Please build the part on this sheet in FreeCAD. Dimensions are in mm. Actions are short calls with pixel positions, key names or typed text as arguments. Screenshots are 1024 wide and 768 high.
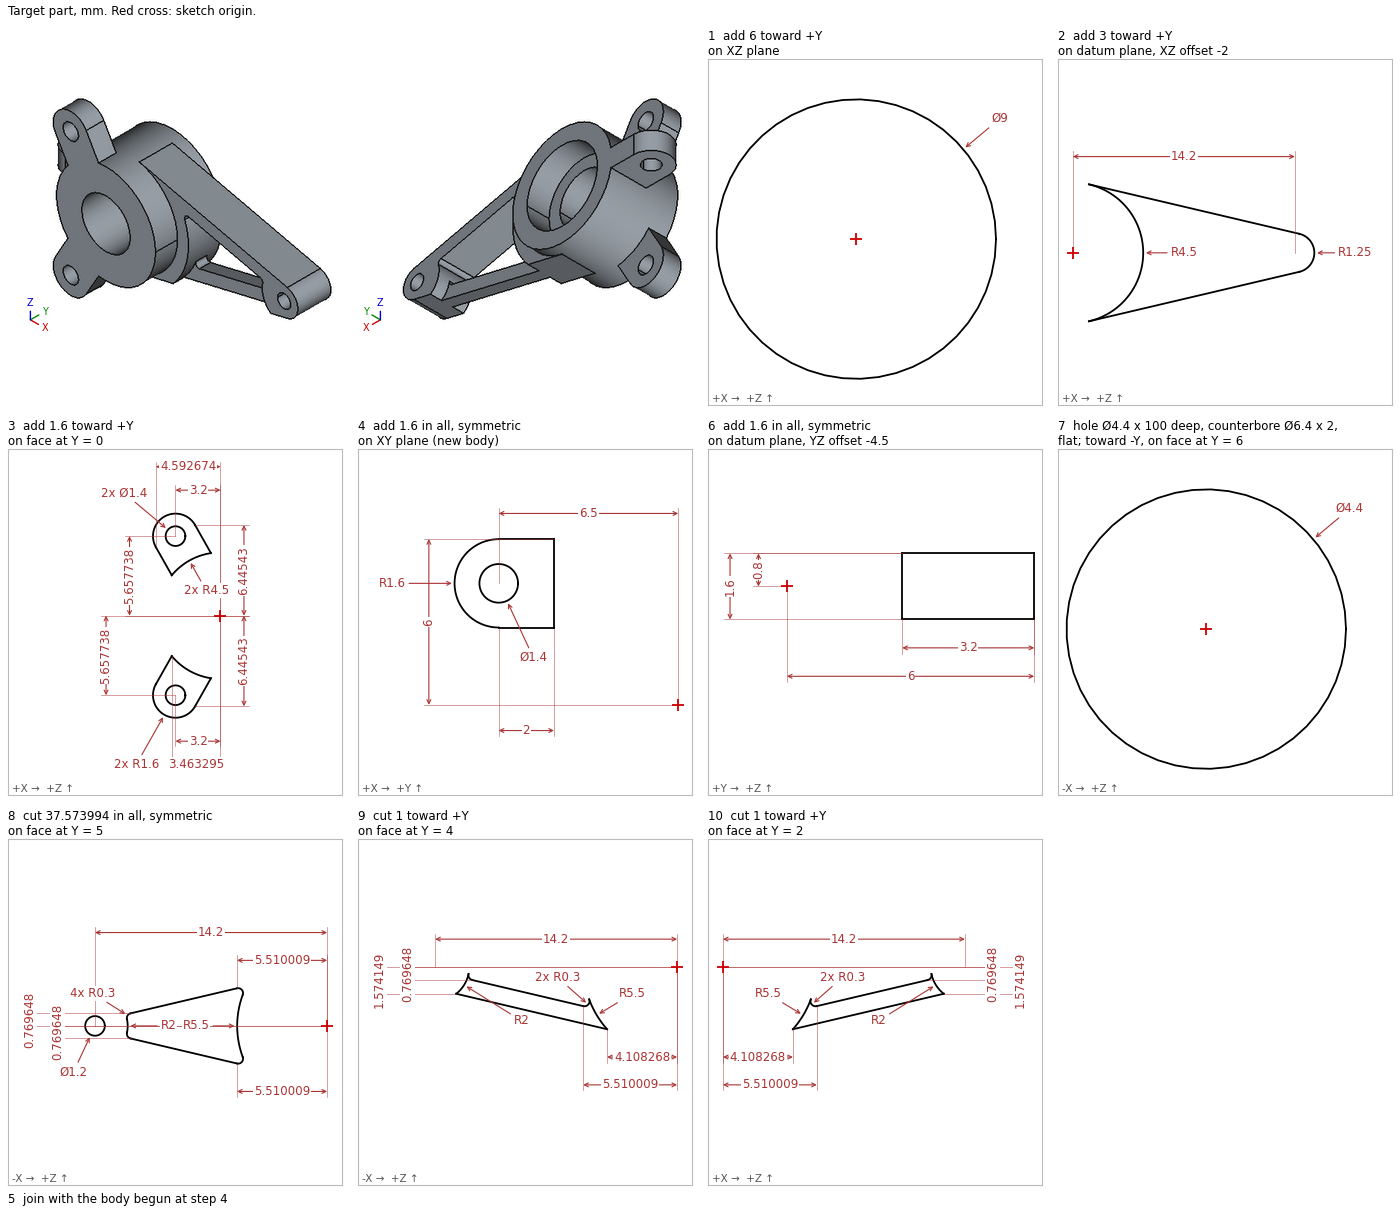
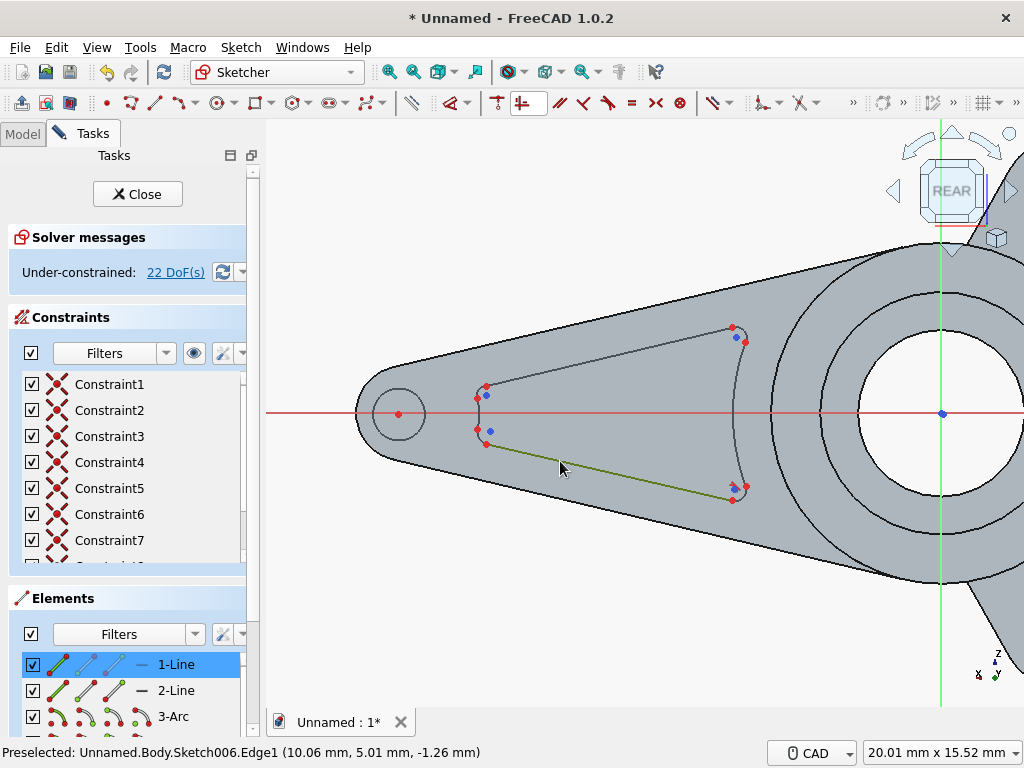
scroll(480, 439, up, 3)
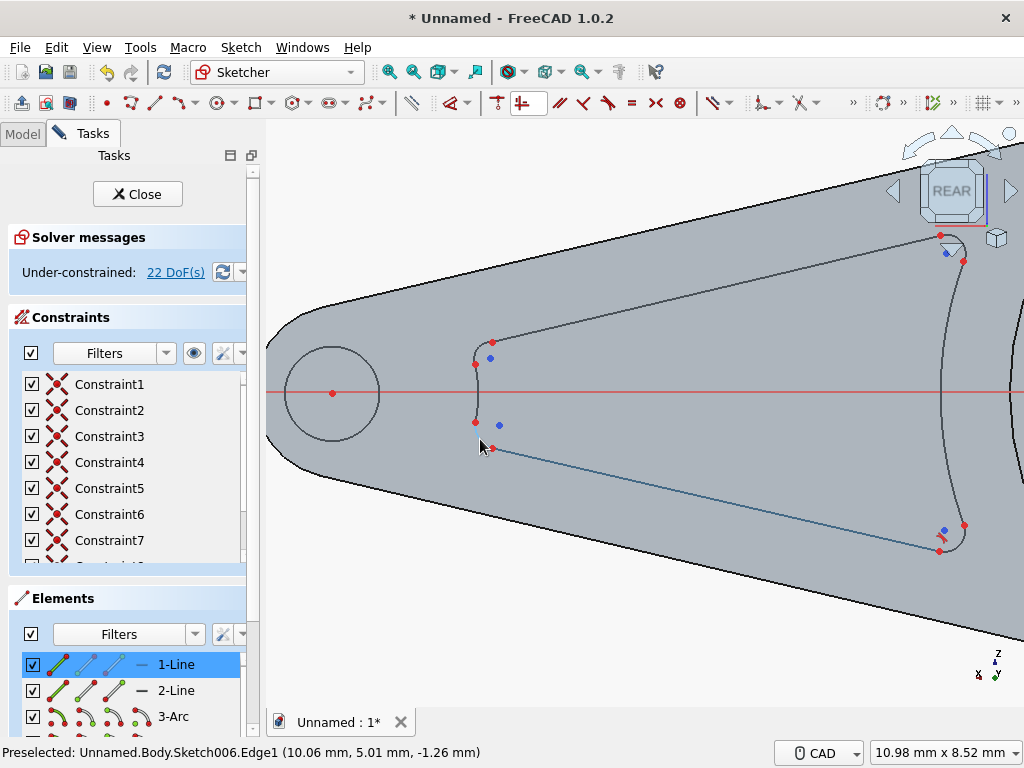
click(479, 438)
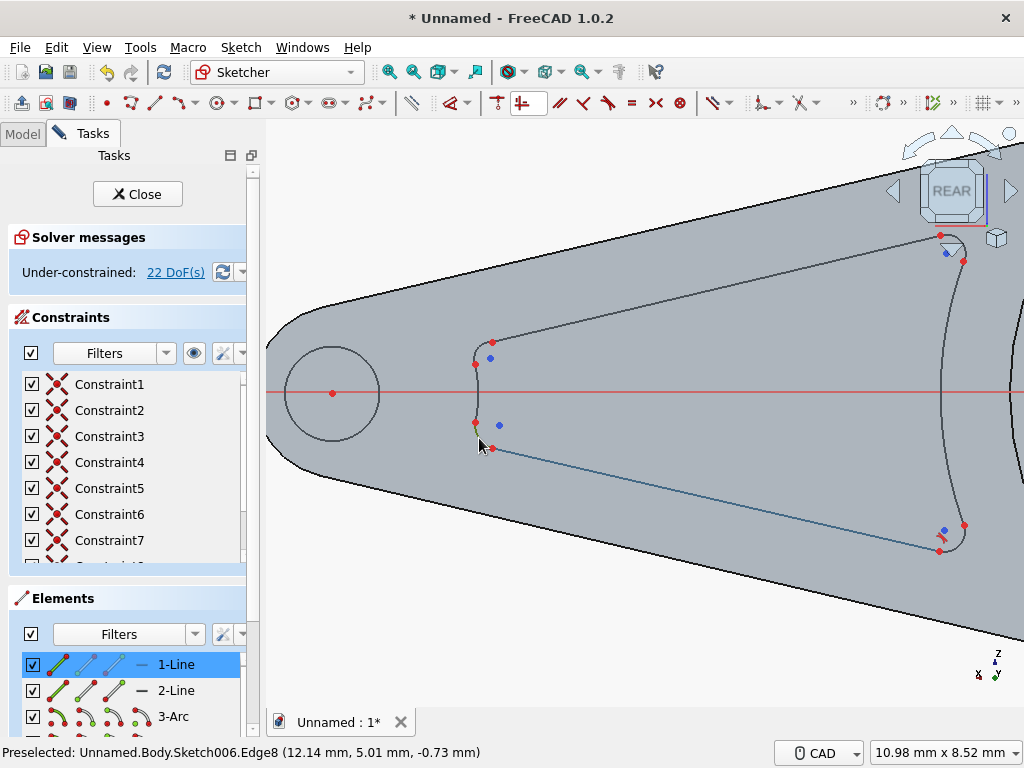
key(t)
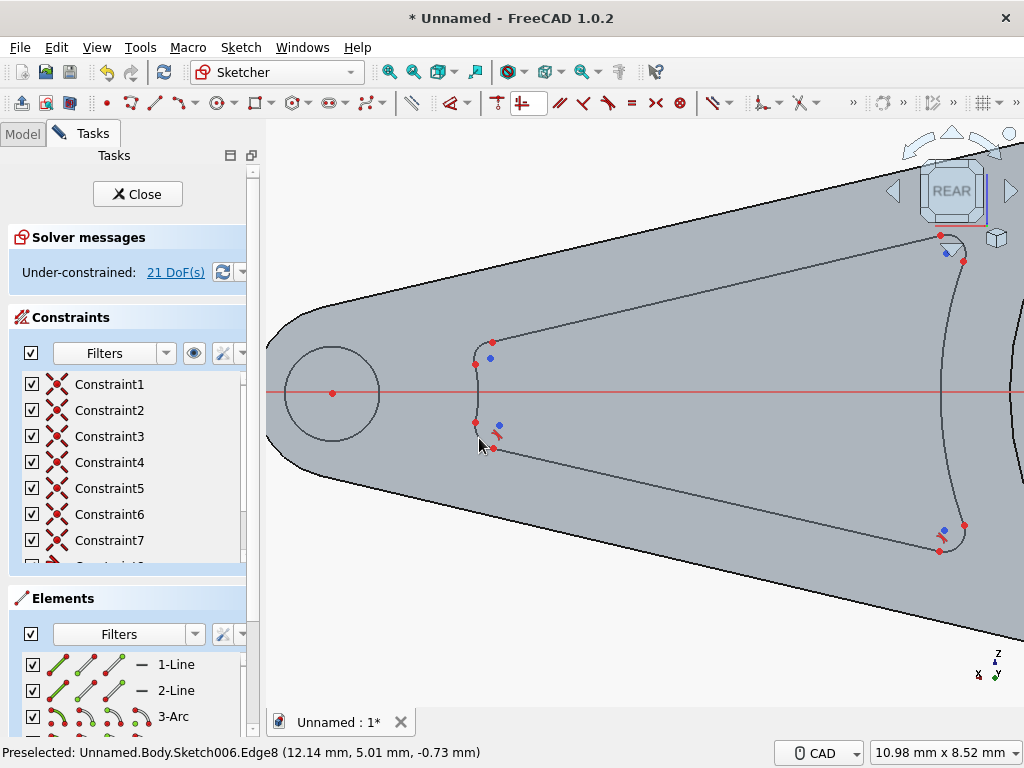
click(806, 268)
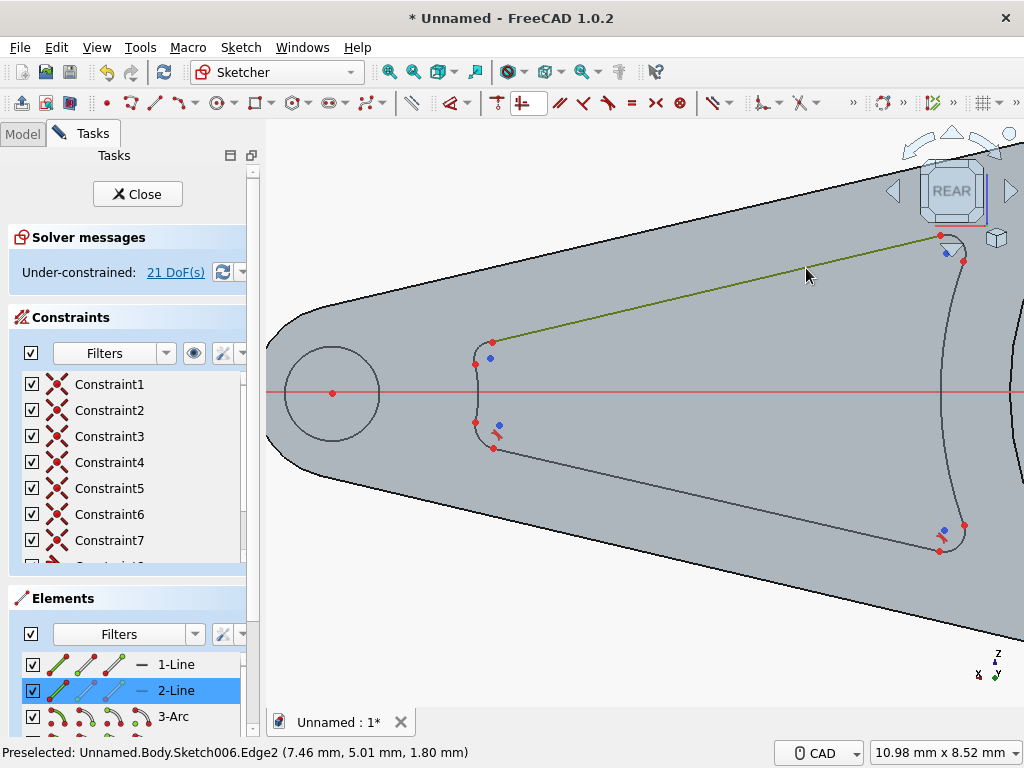
scroll(441, 425, down, 5)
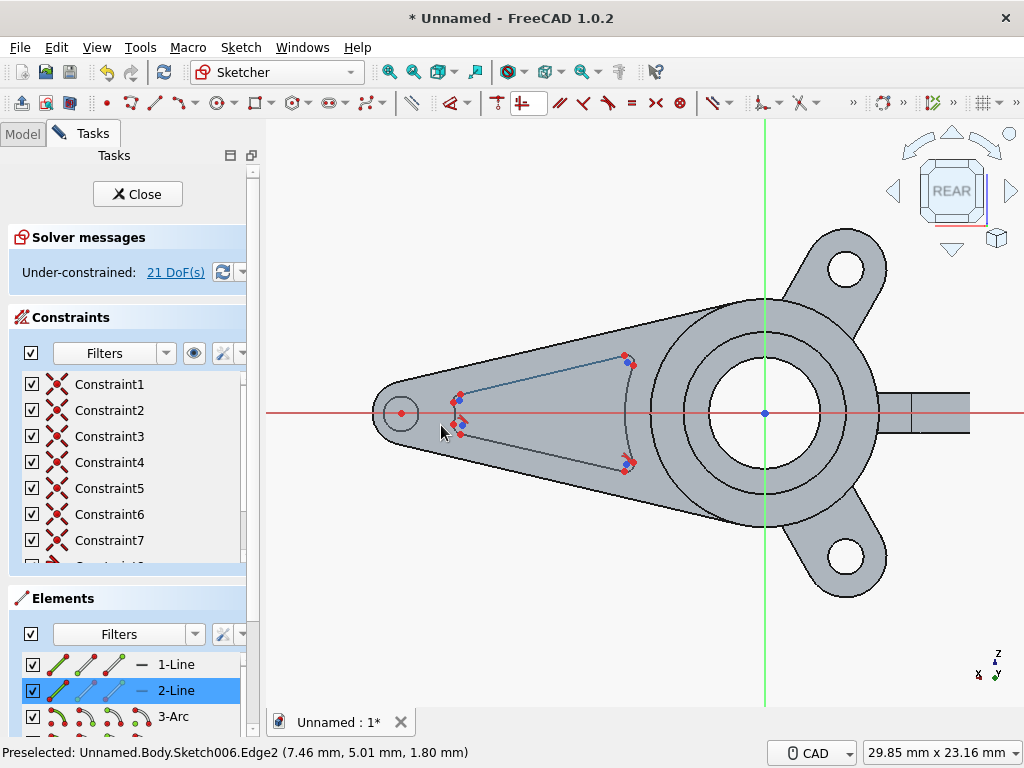
scroll(634, 361, up, 6)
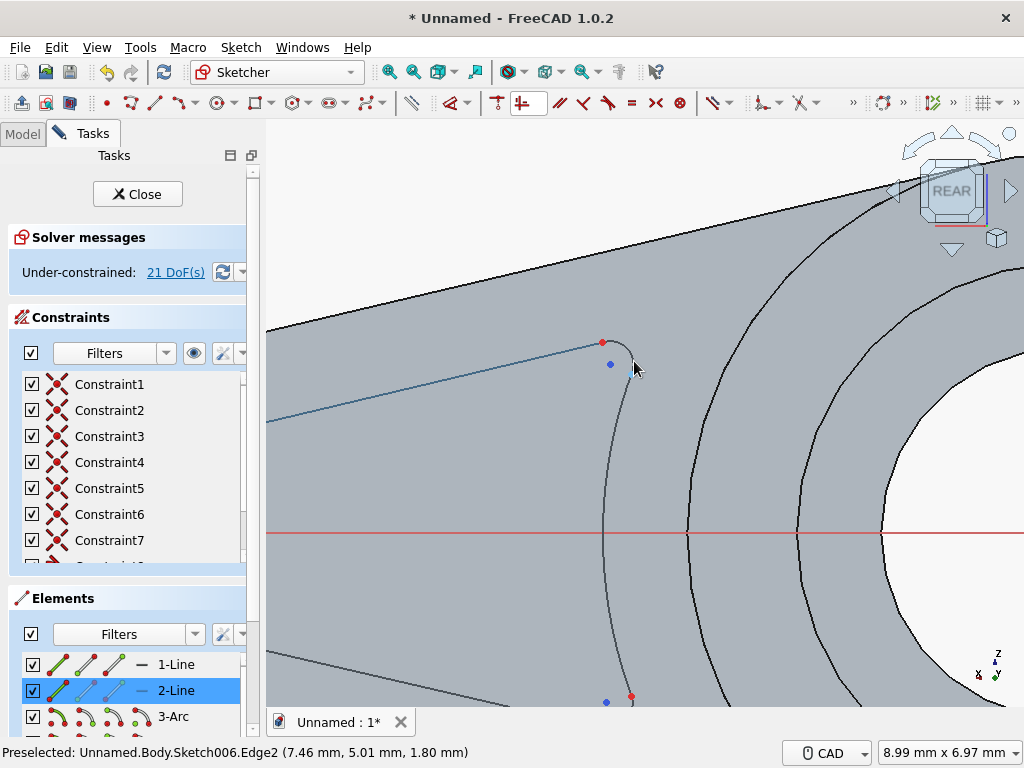
click(633, 359)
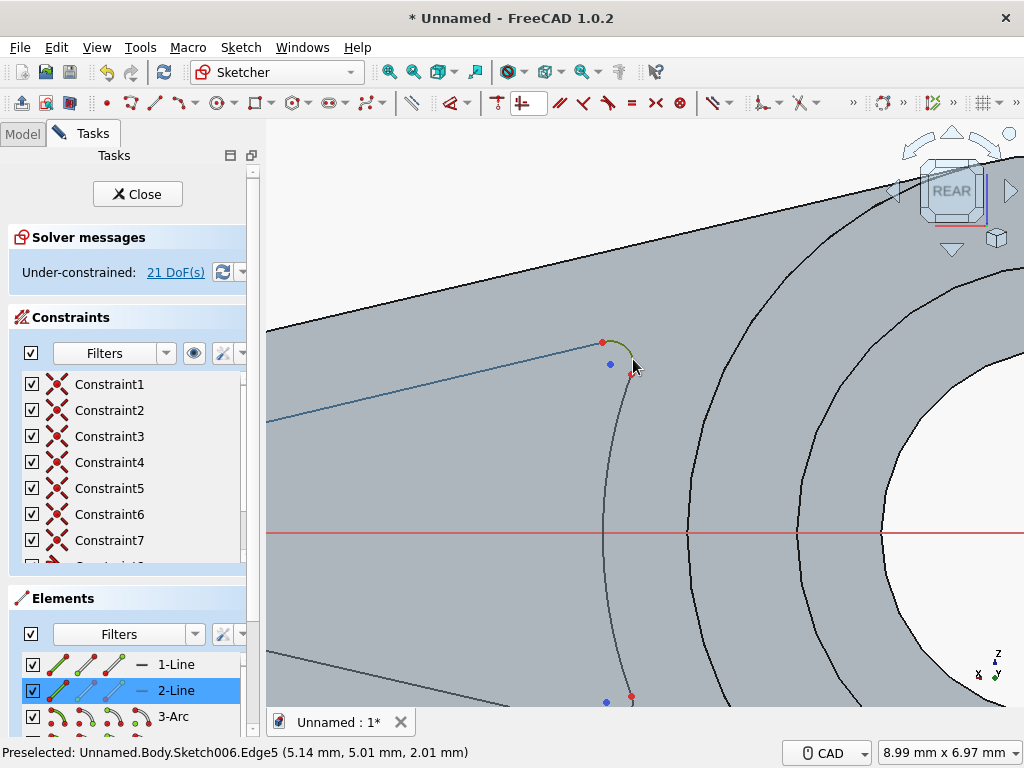
click(608, 104)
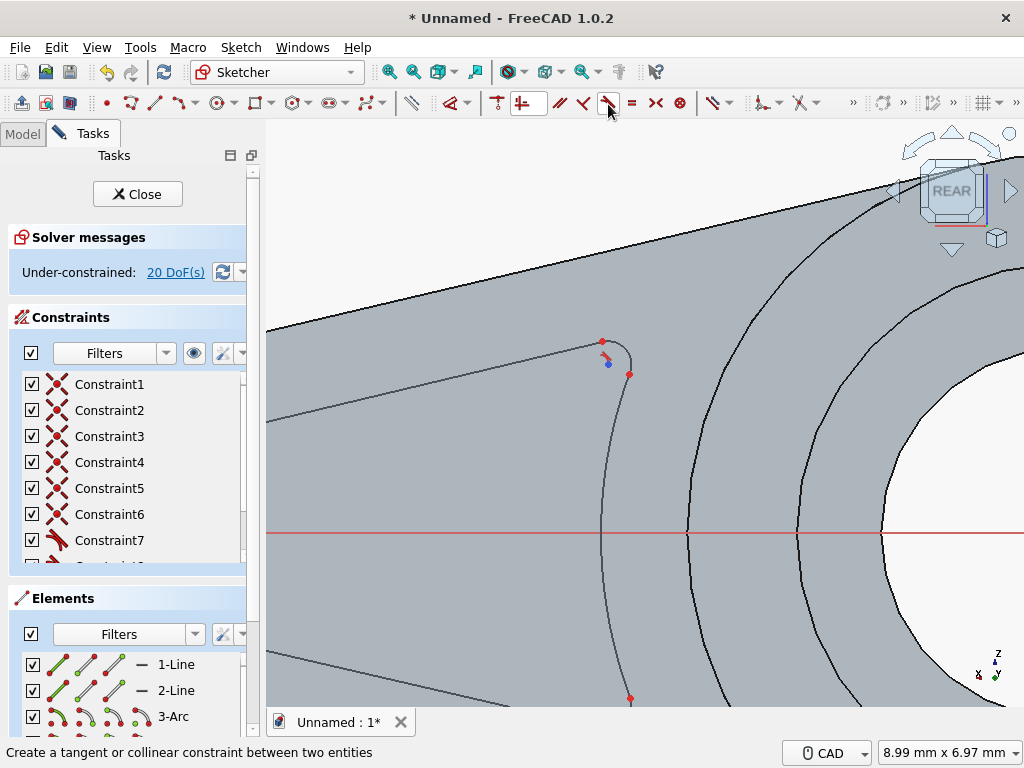
scroll(634, 361, down, 6)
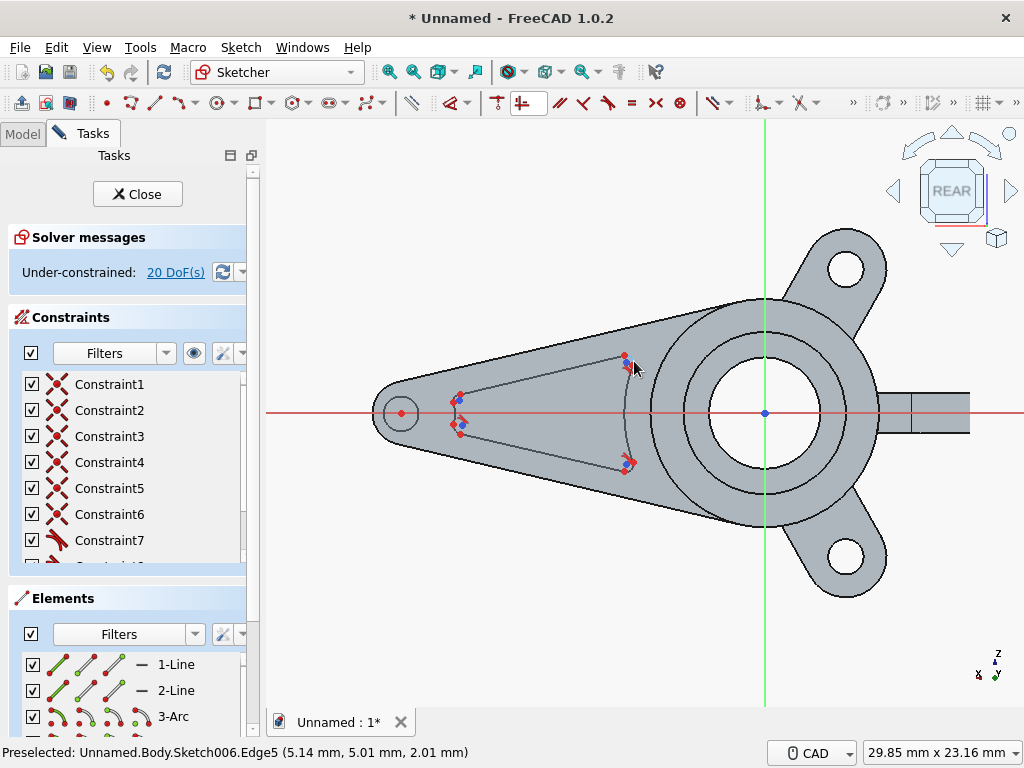
click(575, 367)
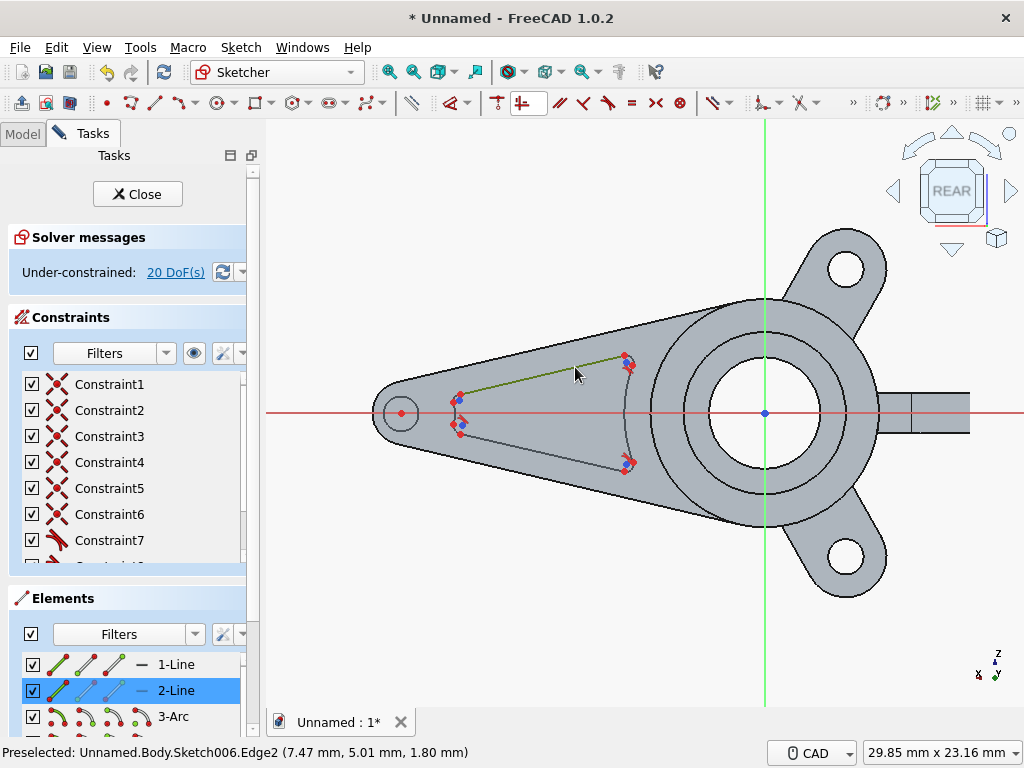
scroll(455, 397, up, 5)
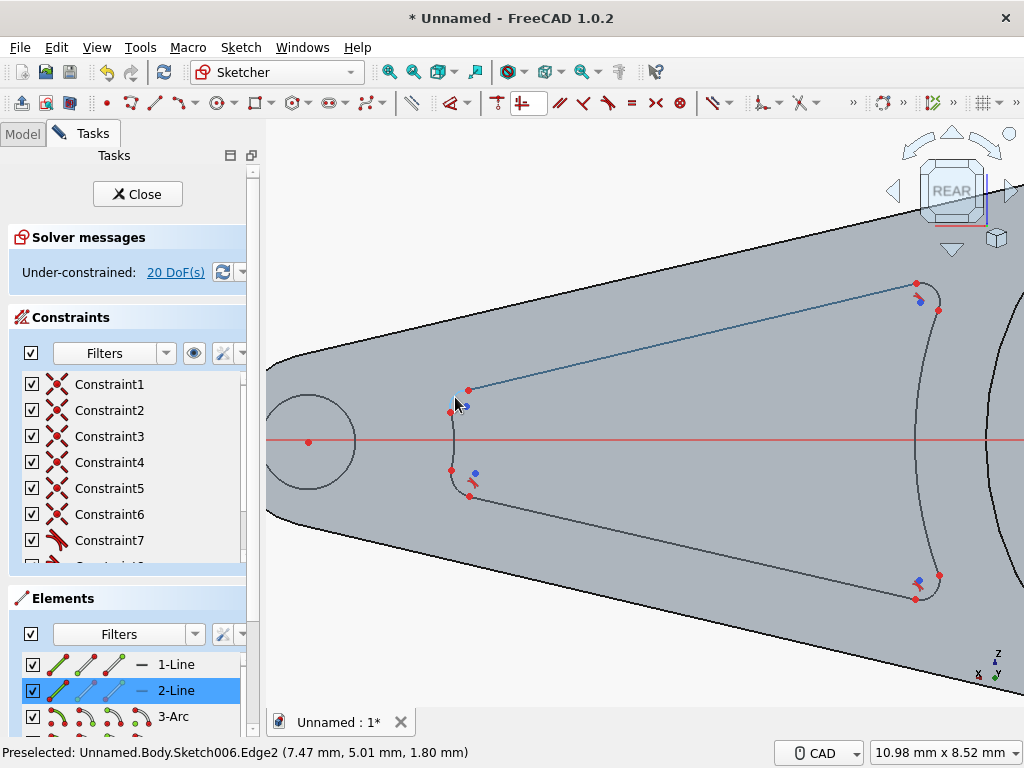
click(454, 397)